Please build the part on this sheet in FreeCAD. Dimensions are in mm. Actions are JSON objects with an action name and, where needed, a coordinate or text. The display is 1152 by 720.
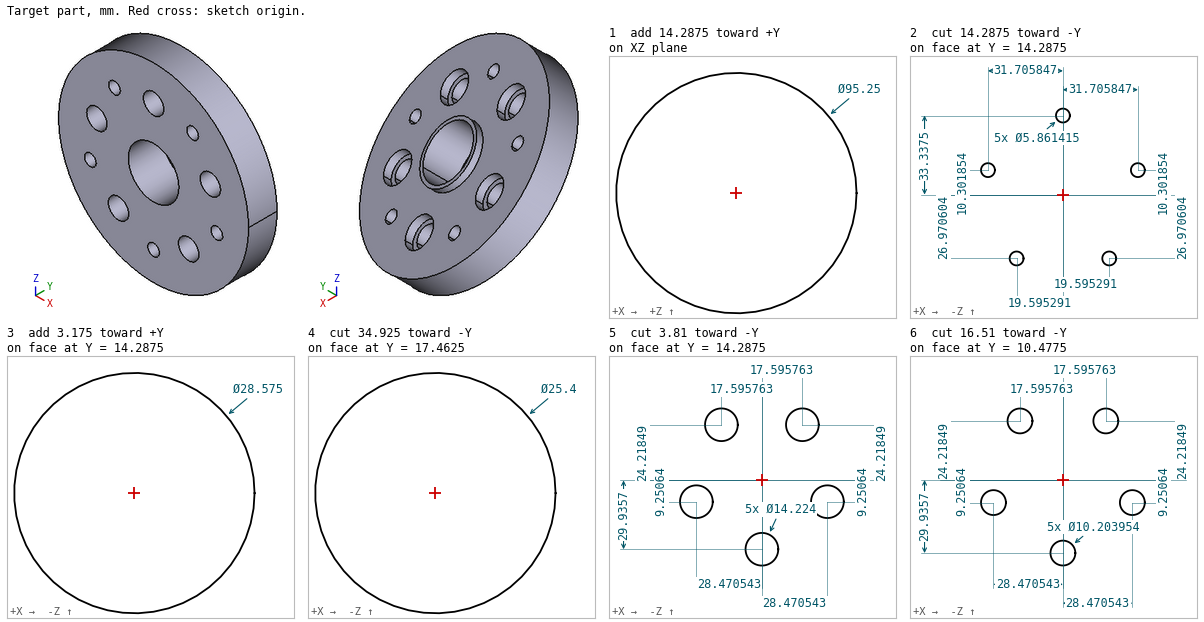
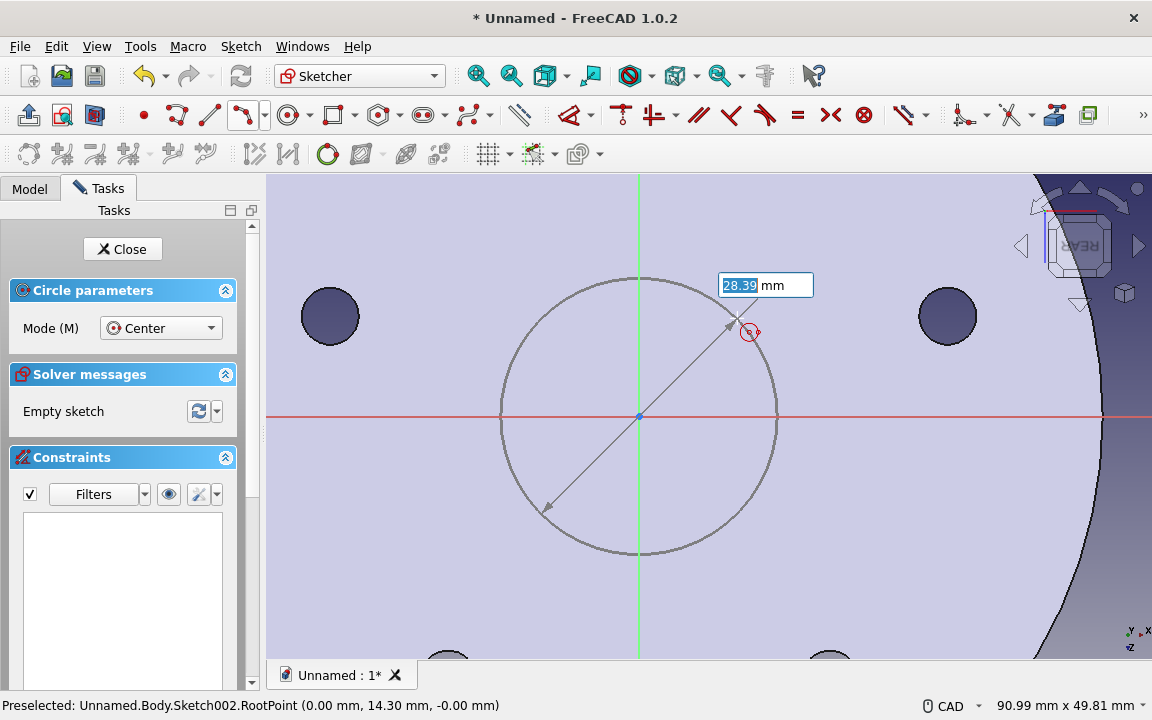
{"action": "type", "text": "28.575"}
{"action": "key", "text": "Return"}
{"action": "key", "text": "Escape"}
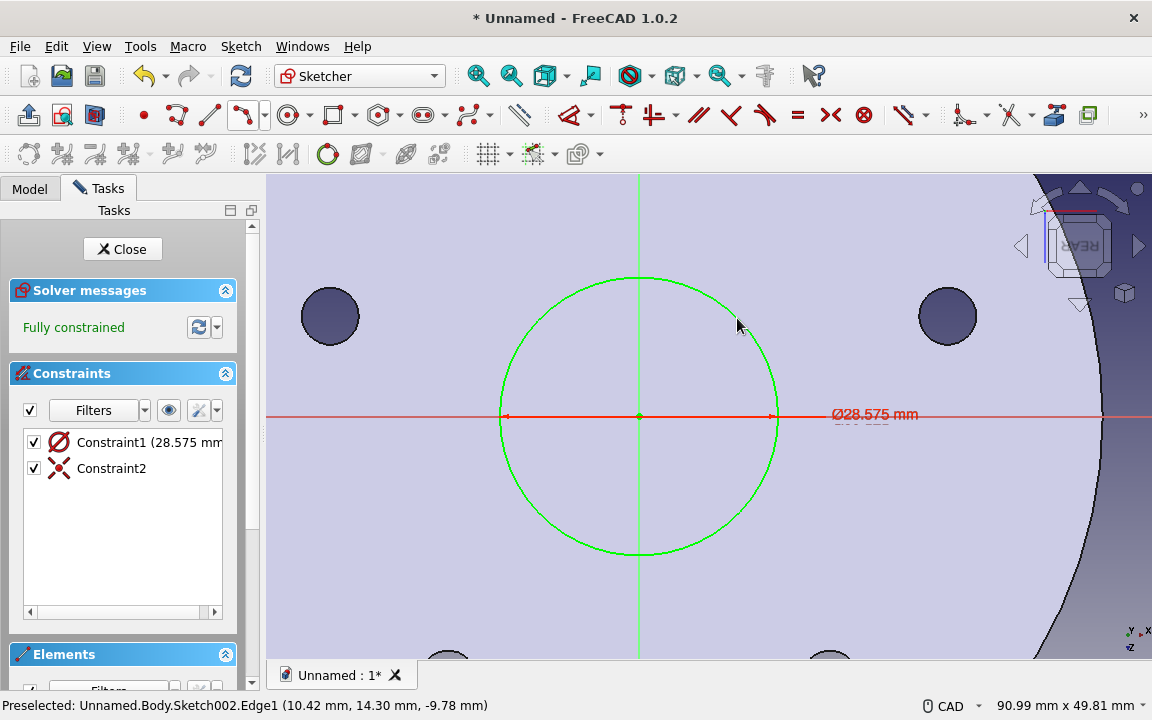
{"action": "left_click", "coordinate": [123, 249]}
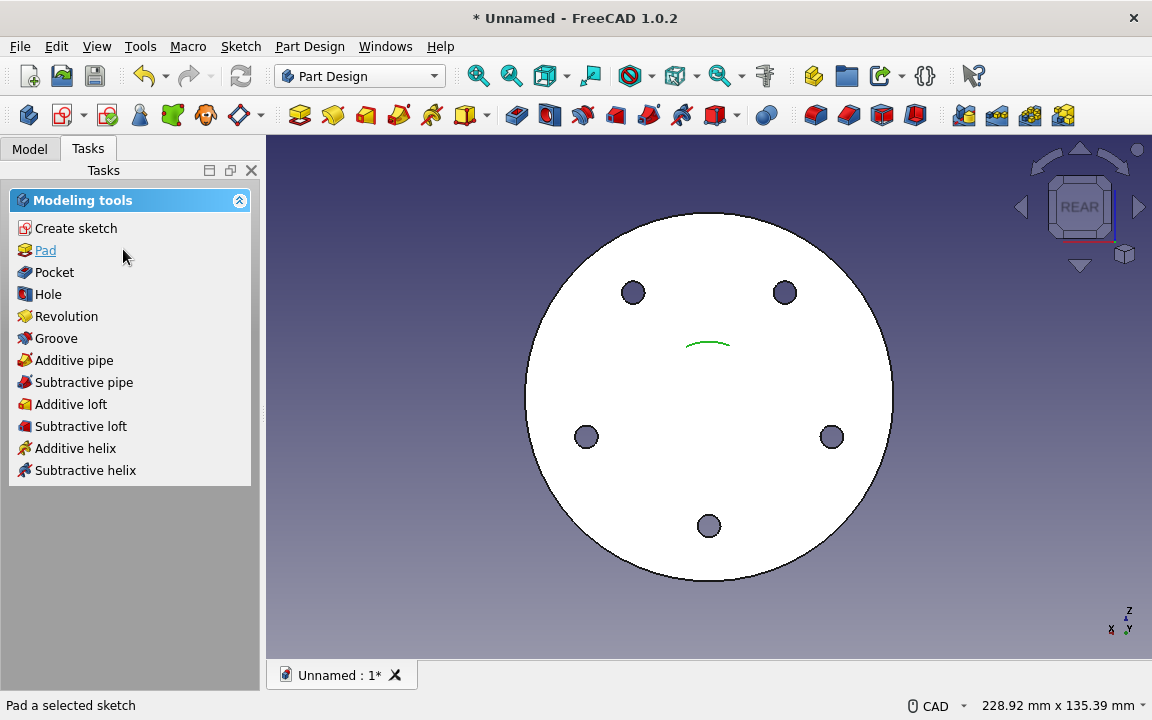
{"action": "left_click", "coordinate": [300, 116]}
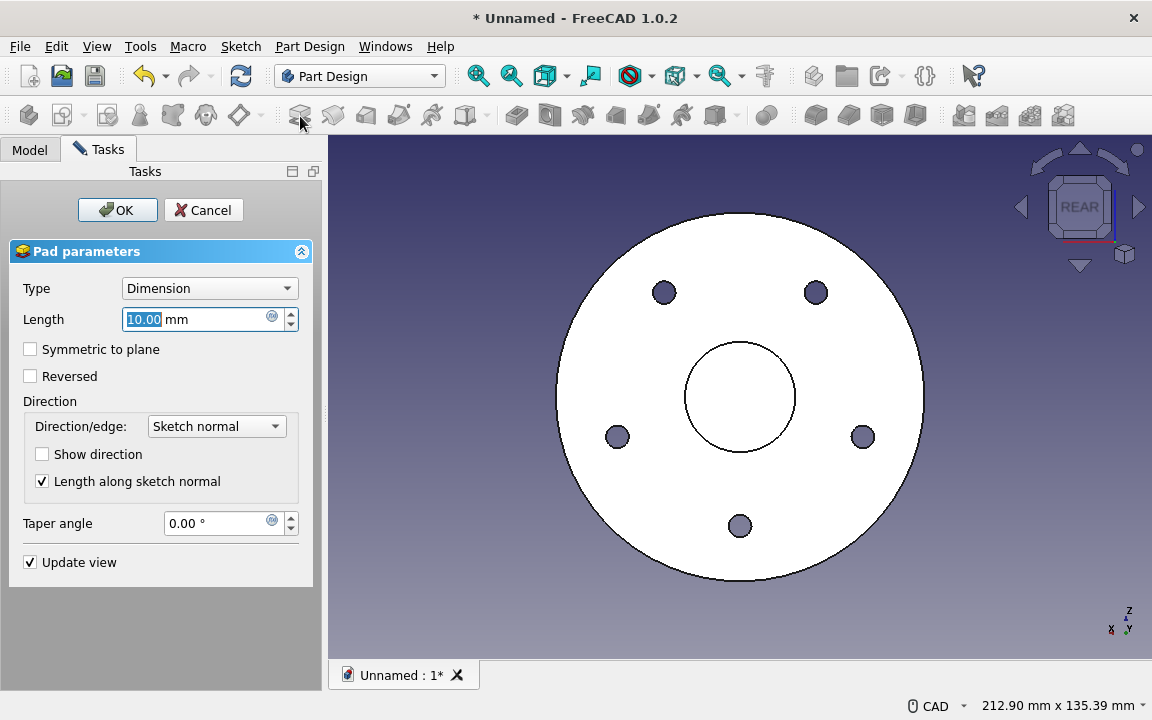
{"action": "type", "text": "3.175"}
{"action": "key", "text": "Tab"}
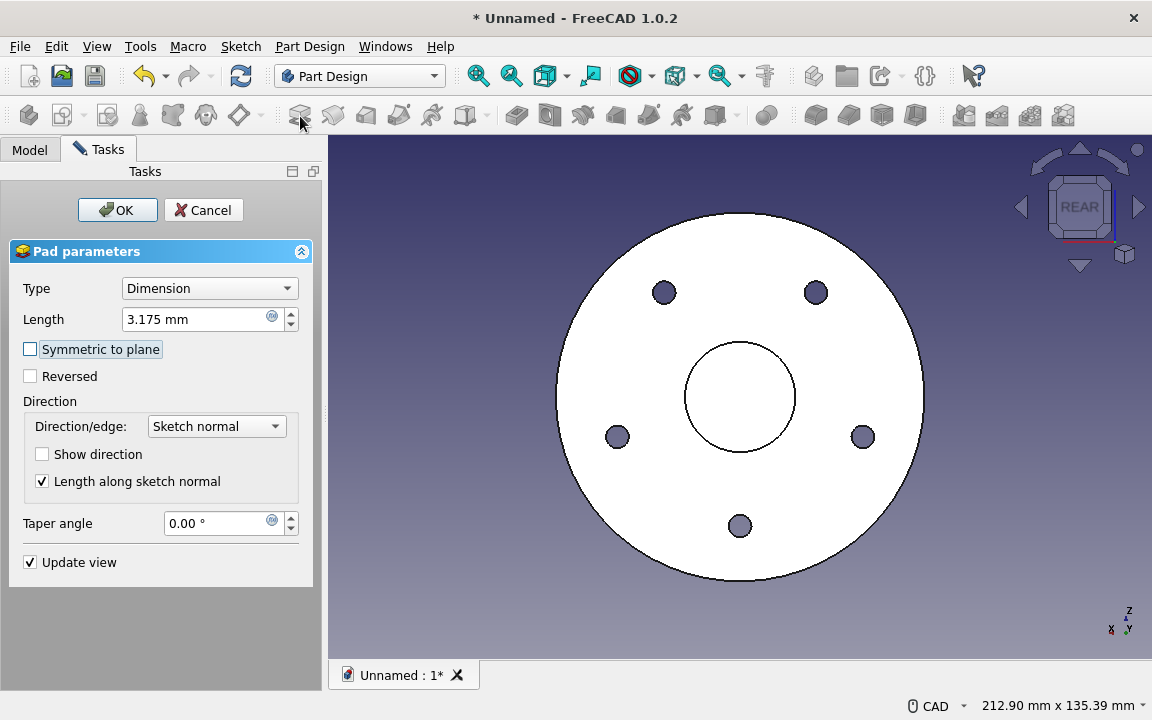
{"action": "left_click", "coordinate": [118, 210]}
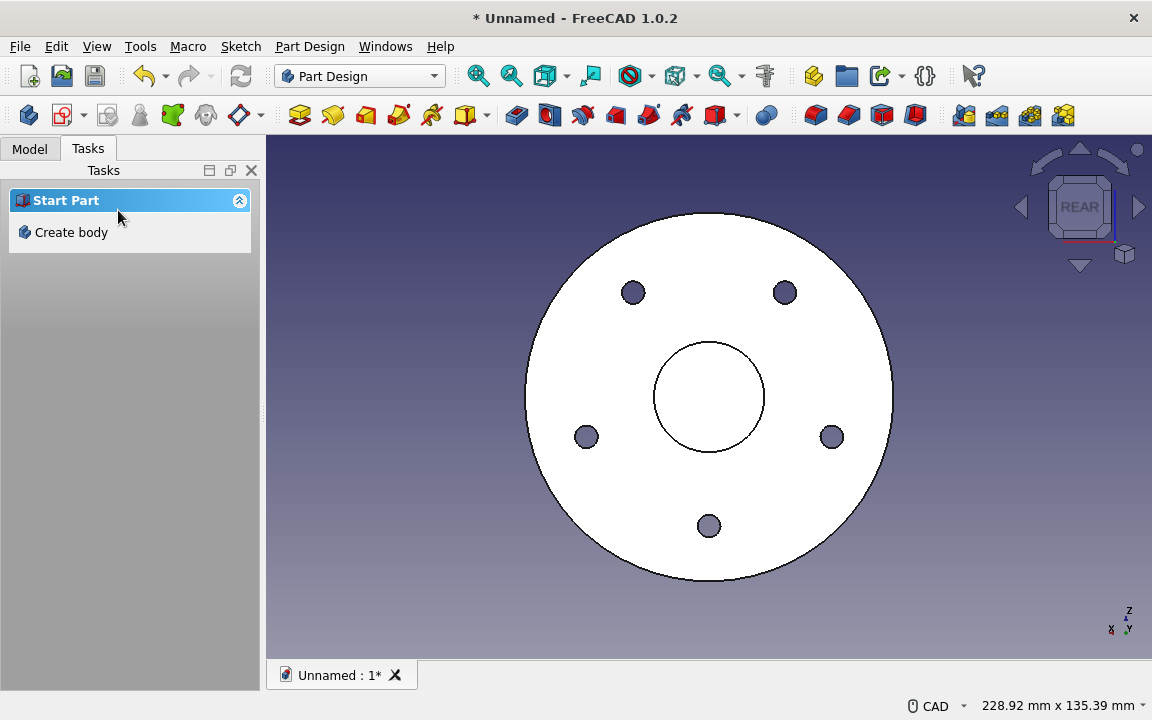
{"action": "left_click", "coordinate": [709, 396]}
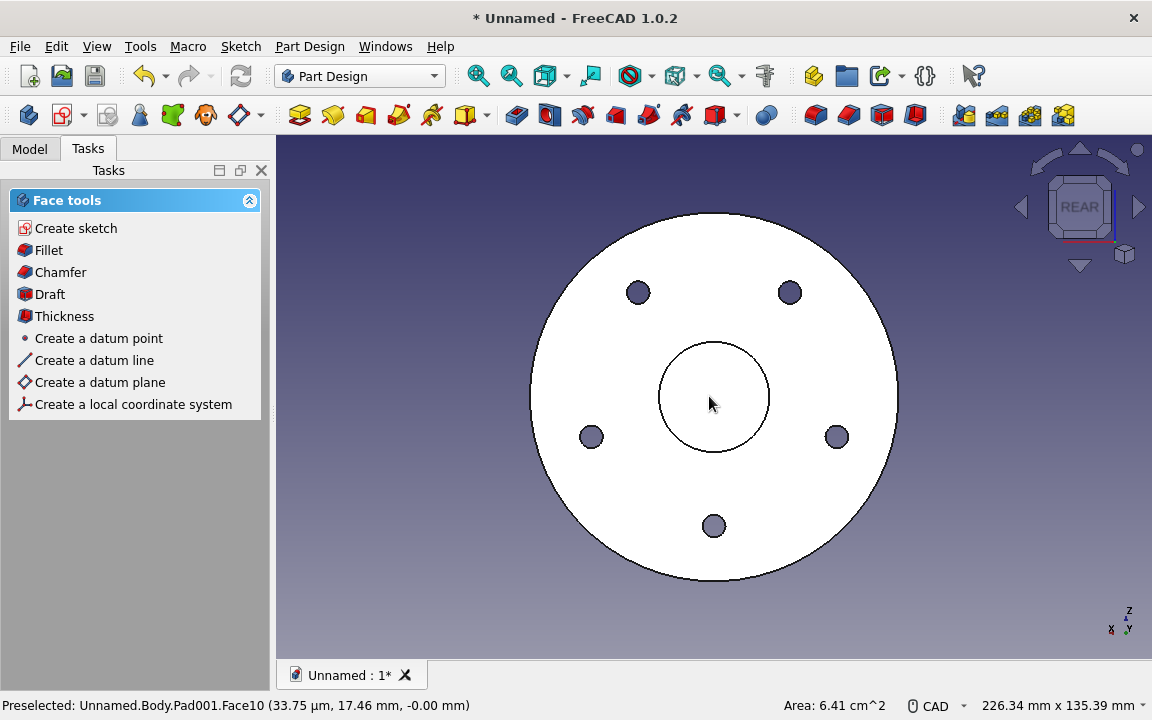
{"action": "left_click", "coordinate": [62, 116]}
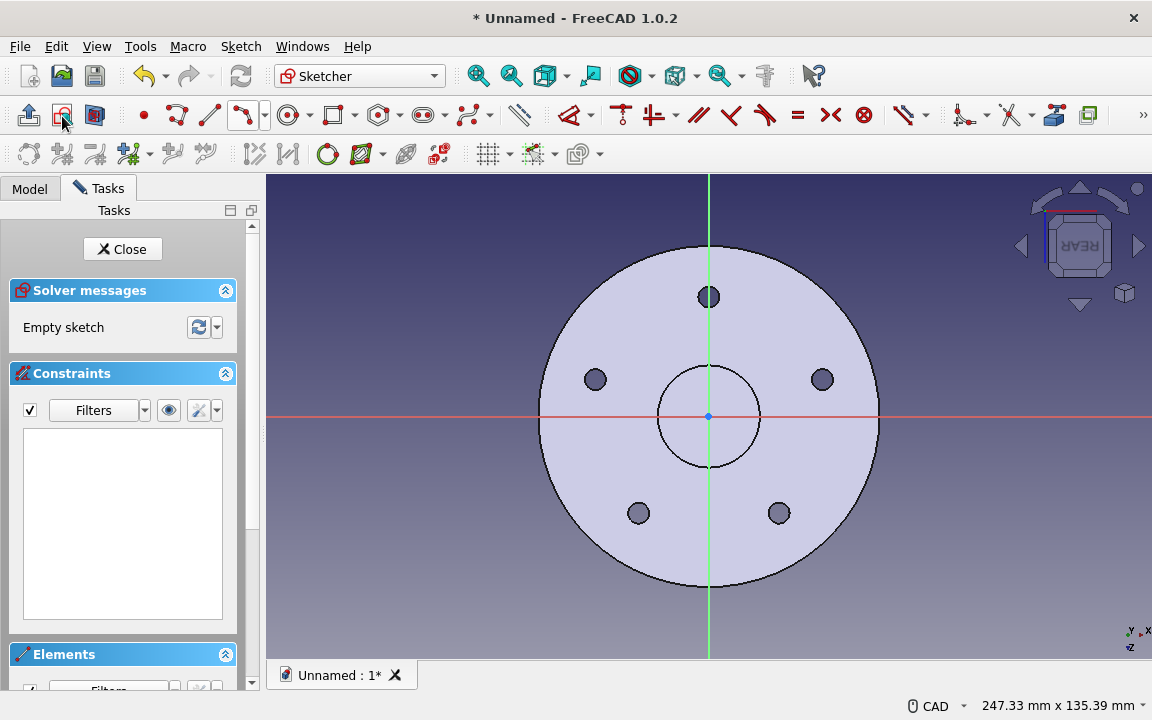
{"action": "scroll", "coordinate": [738, 416], "scroll_direction": "up", "scroll_amount": 6}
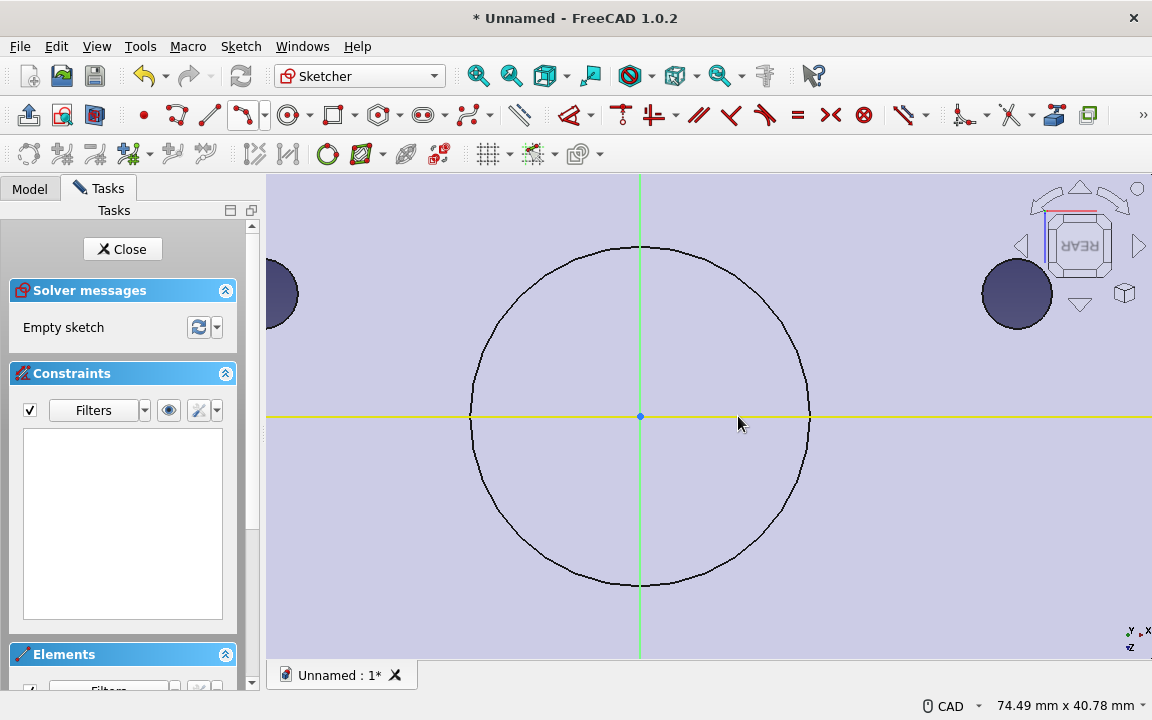
{"action": "left_click", "coordinate": [288, 116]}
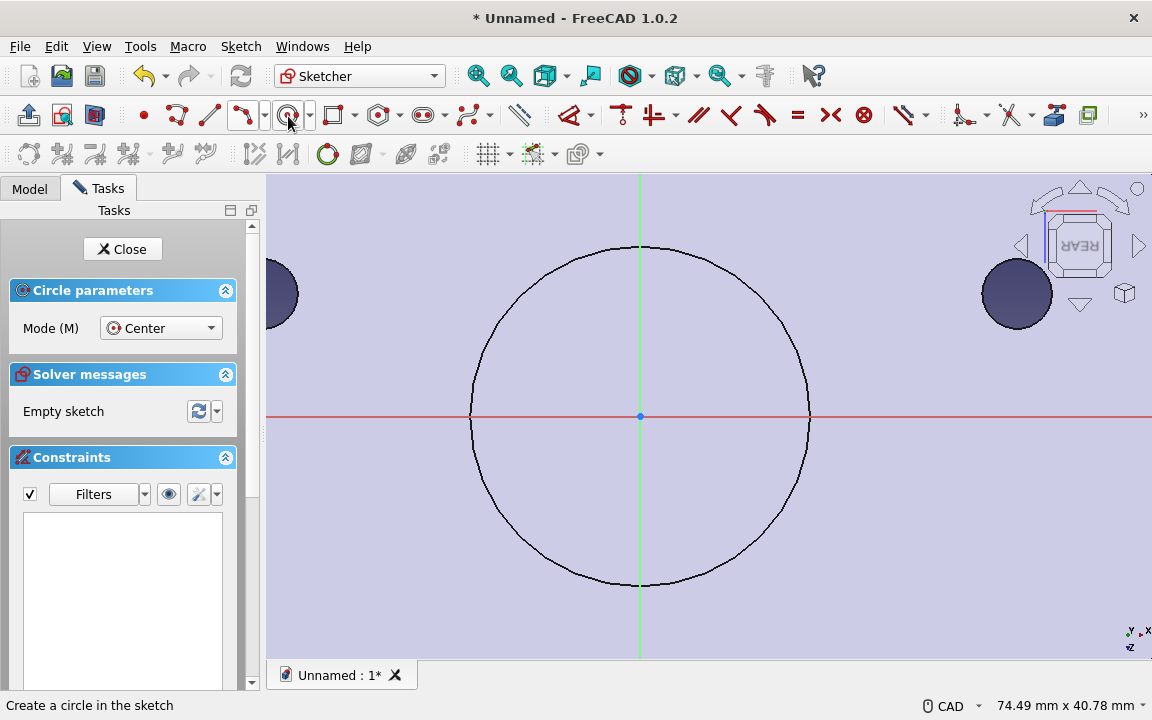
{"action": "left_click", "coordinate": [640, 416]}
{"action": "mouse_move", "coordinate": [747, 310]}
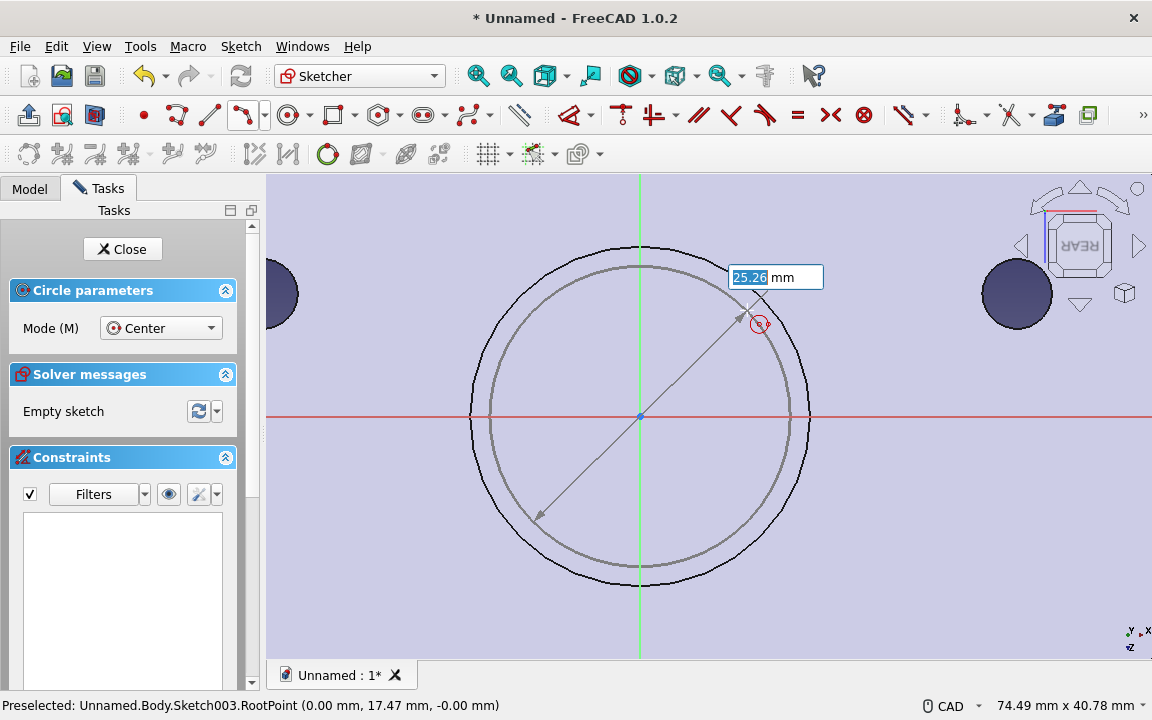
{"action": "type", "text": "25.4"}
{"action": "key", "text": "Return"}
{"action": "key", "text": "Escape"}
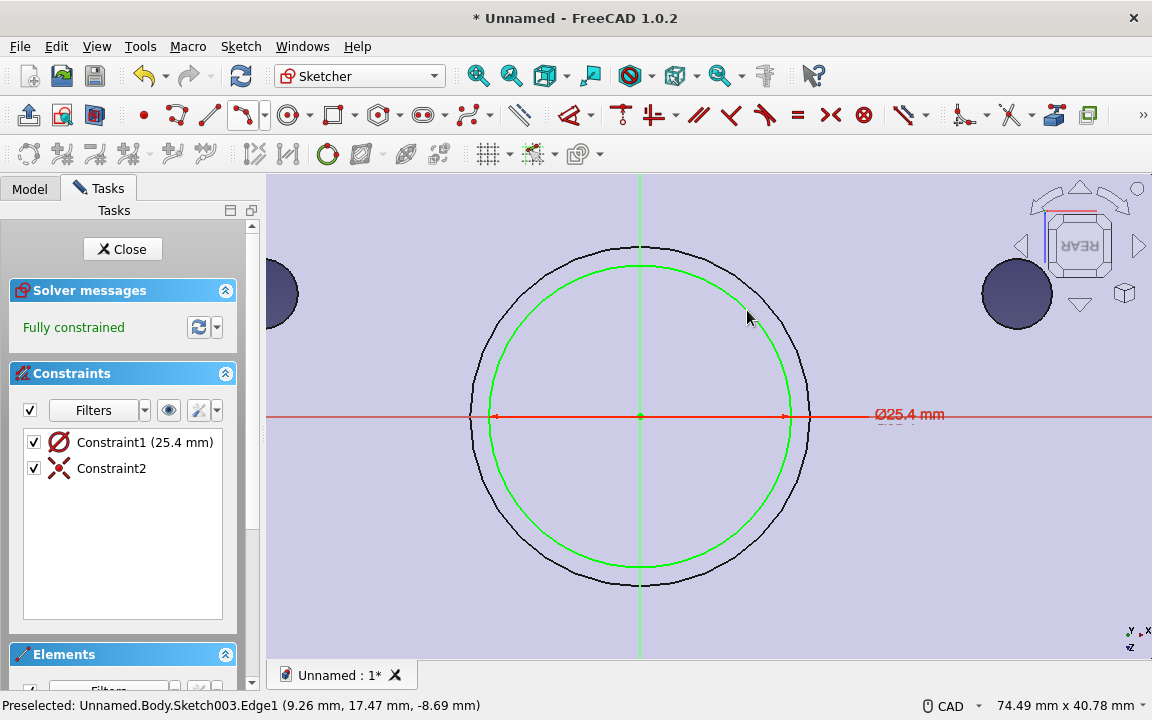
{"action": "left_click", "coordinate": [123, 249]}